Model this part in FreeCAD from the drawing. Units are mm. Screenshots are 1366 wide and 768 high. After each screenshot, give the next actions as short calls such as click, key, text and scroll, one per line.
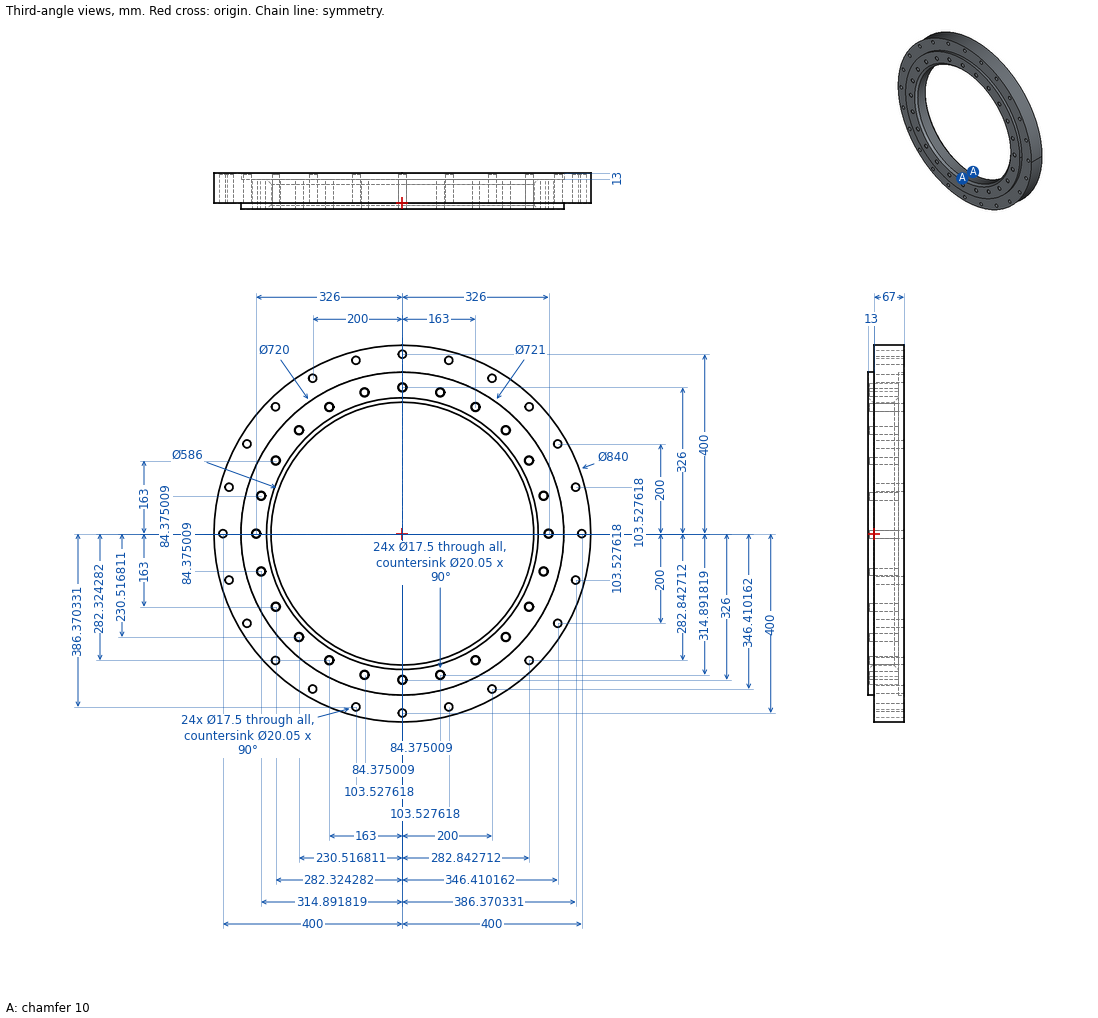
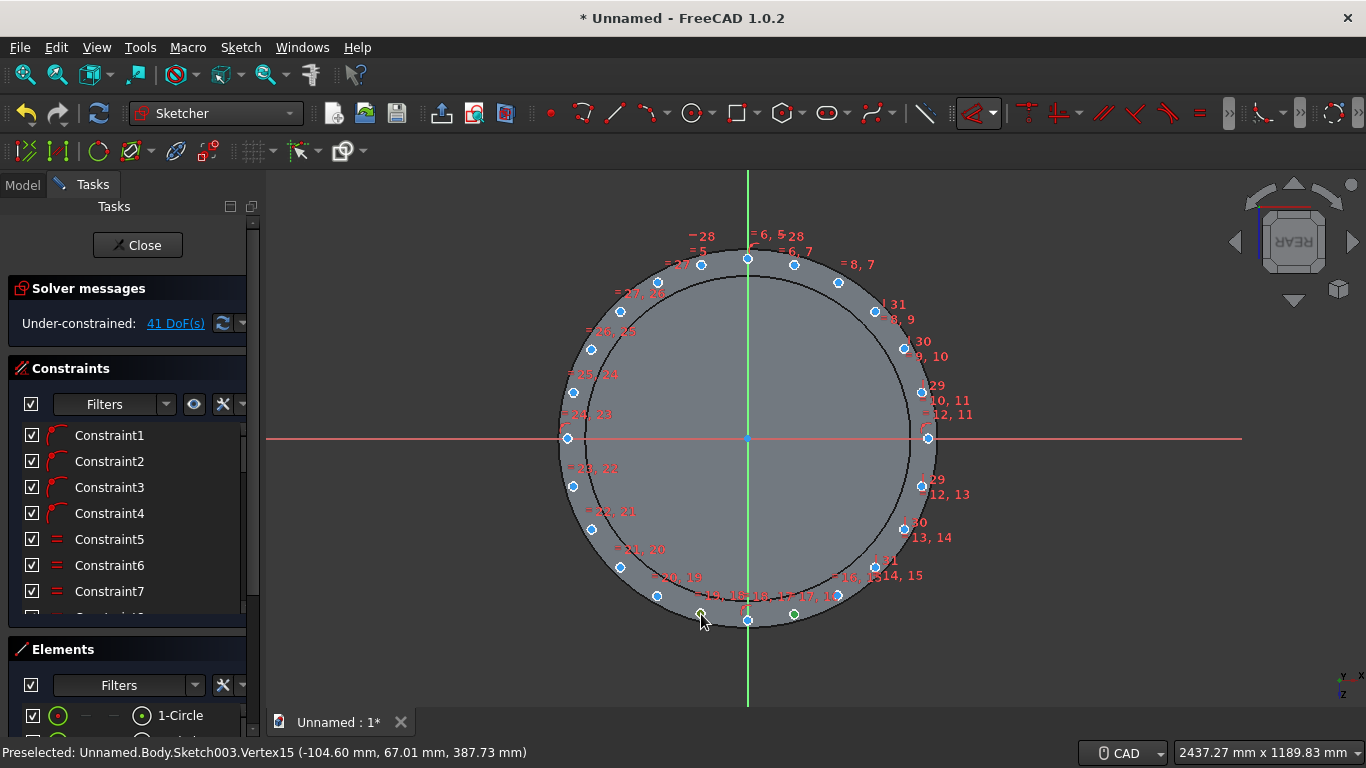
click(1082, 114)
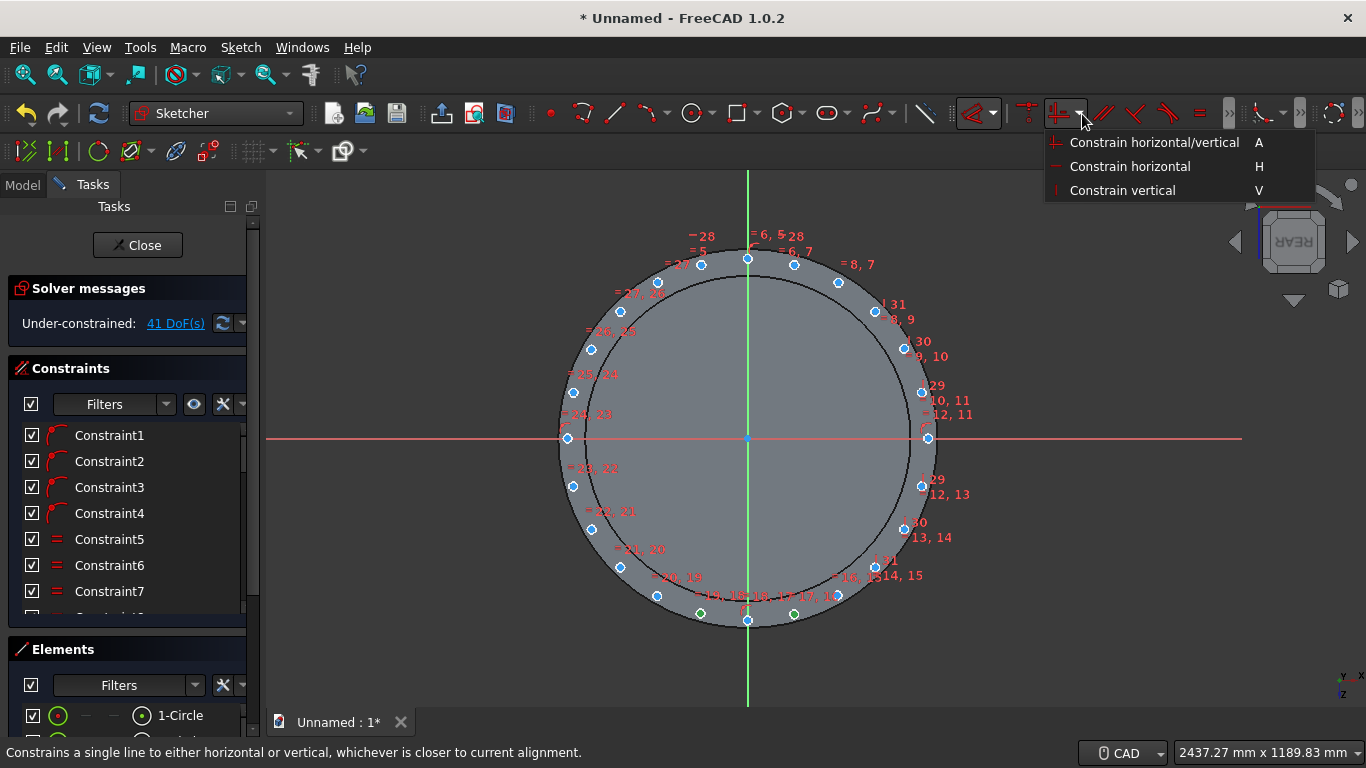
click(1180, 166)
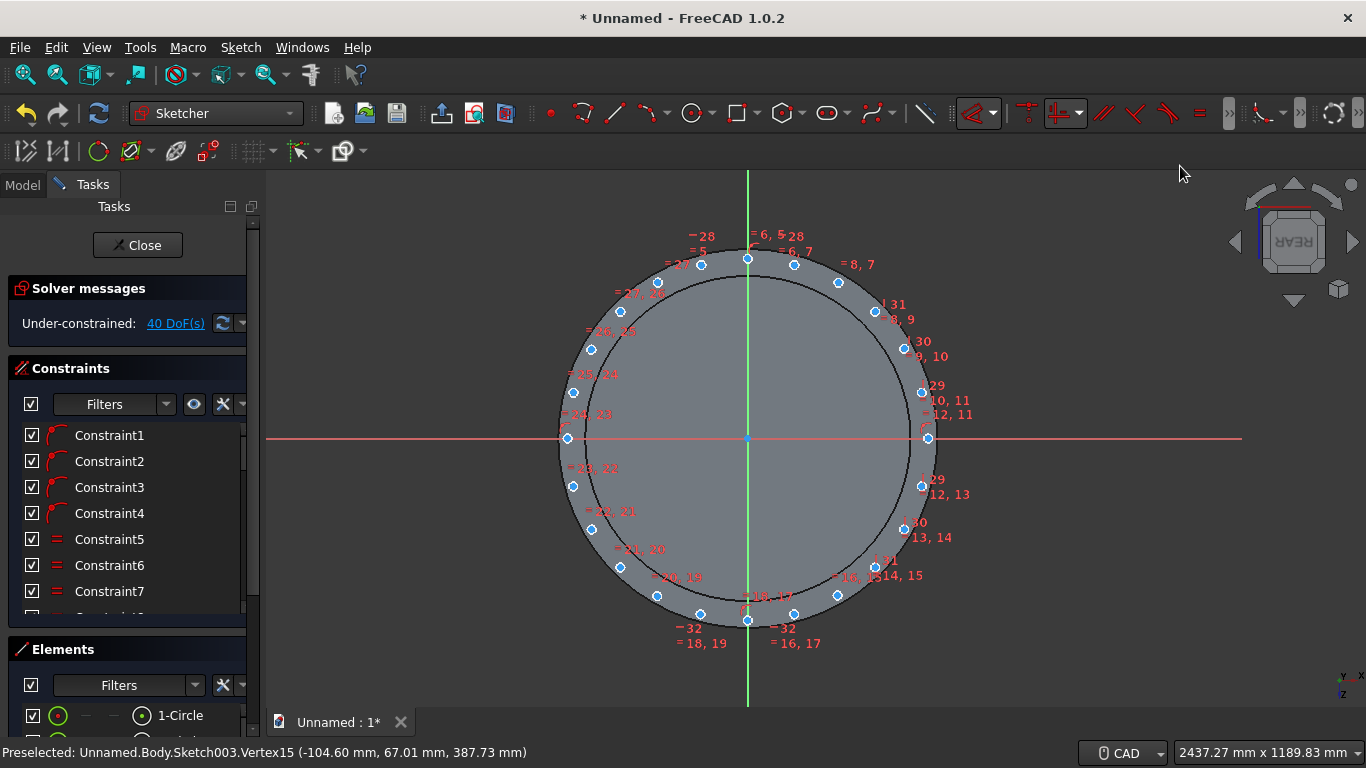
click(838, 596)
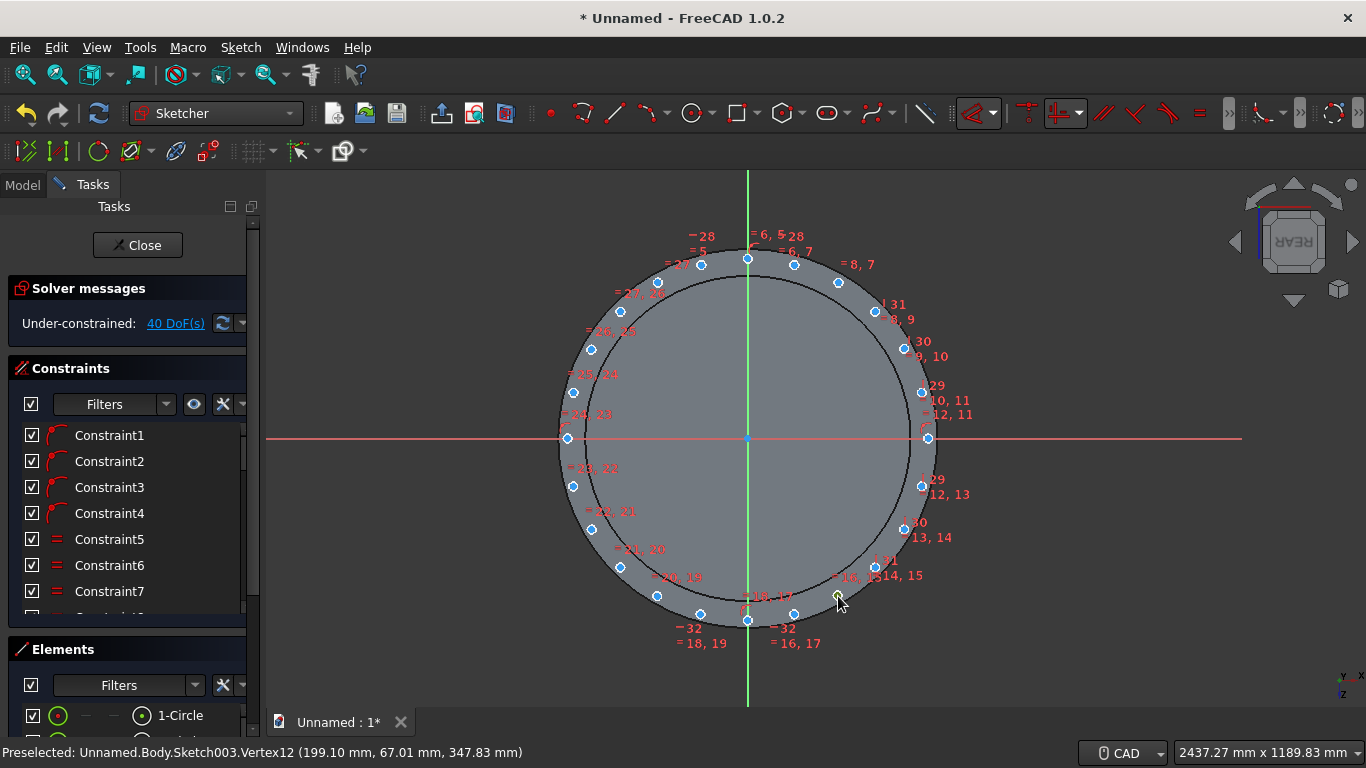
click(657, 596)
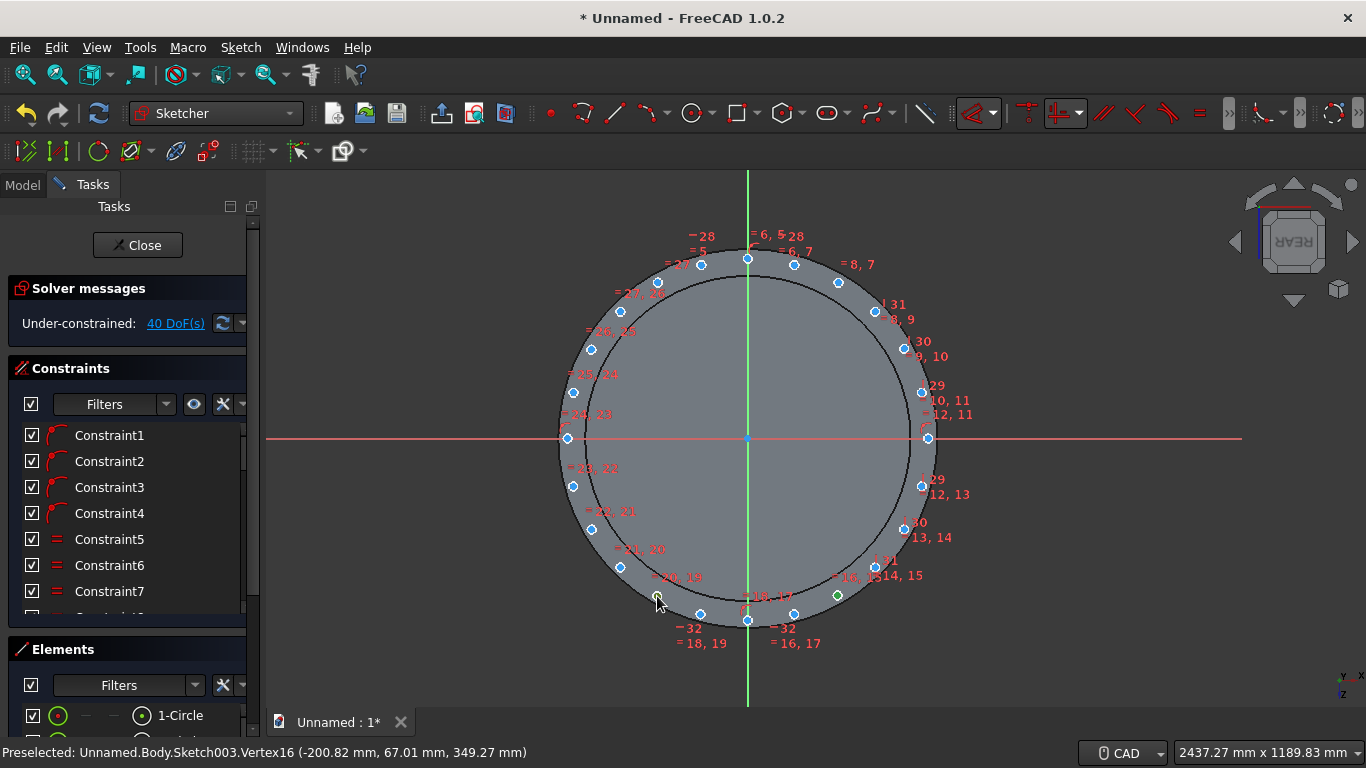
click(1082, 114)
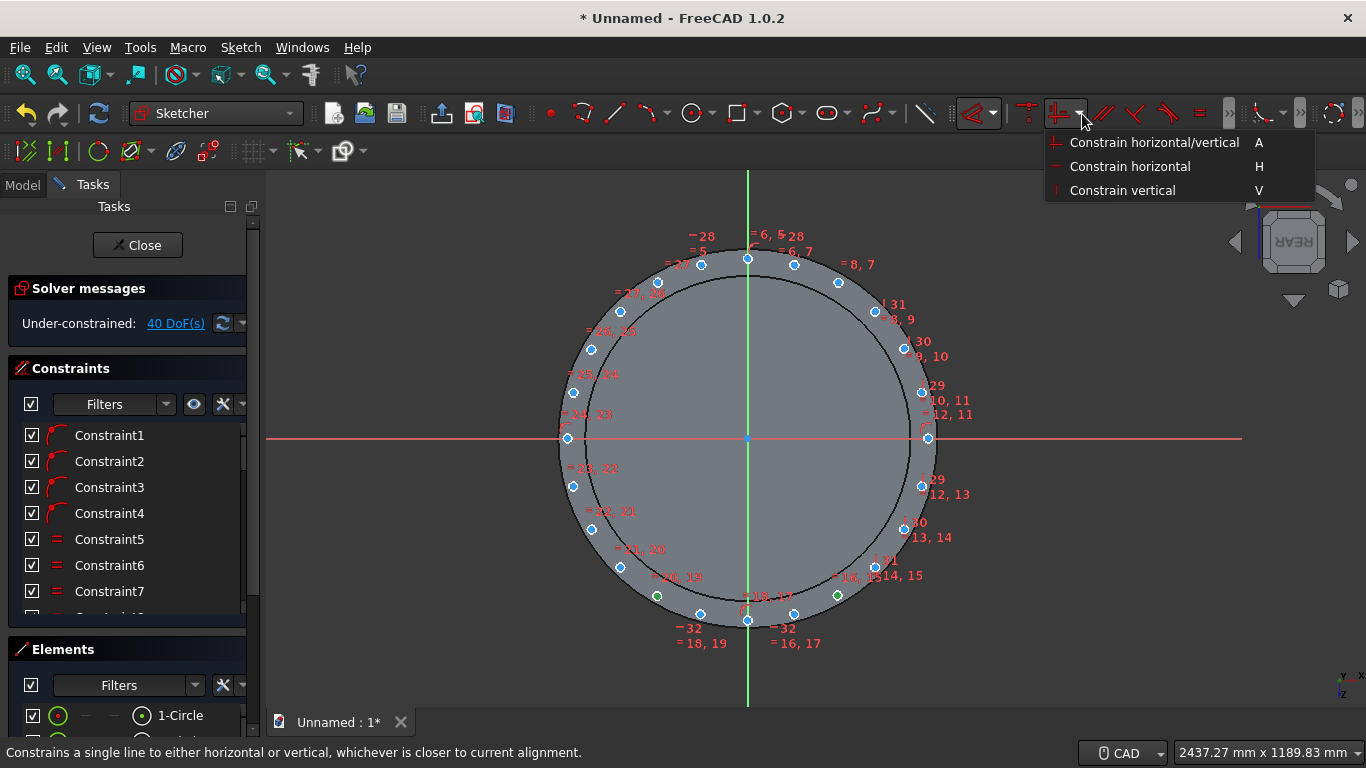
click(1180, 166)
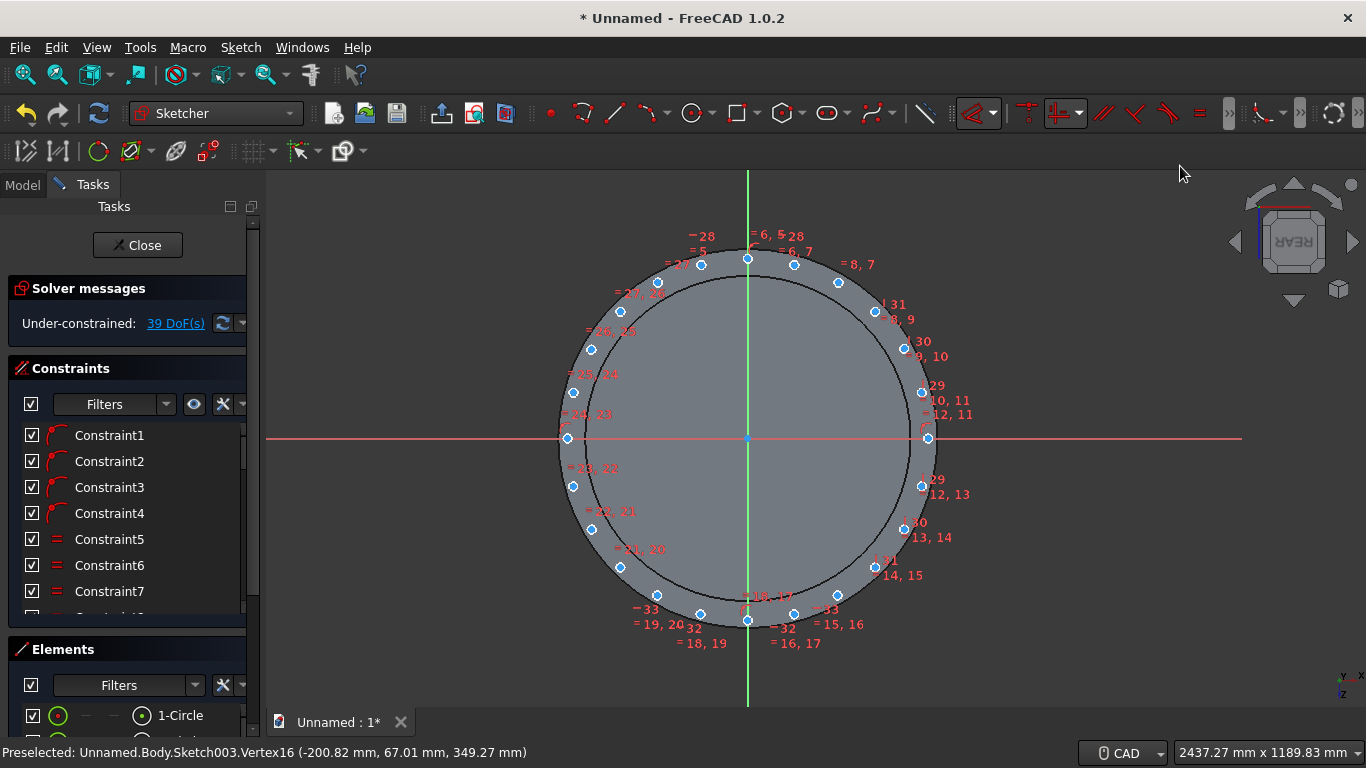
scroll(875, 568, up, 4)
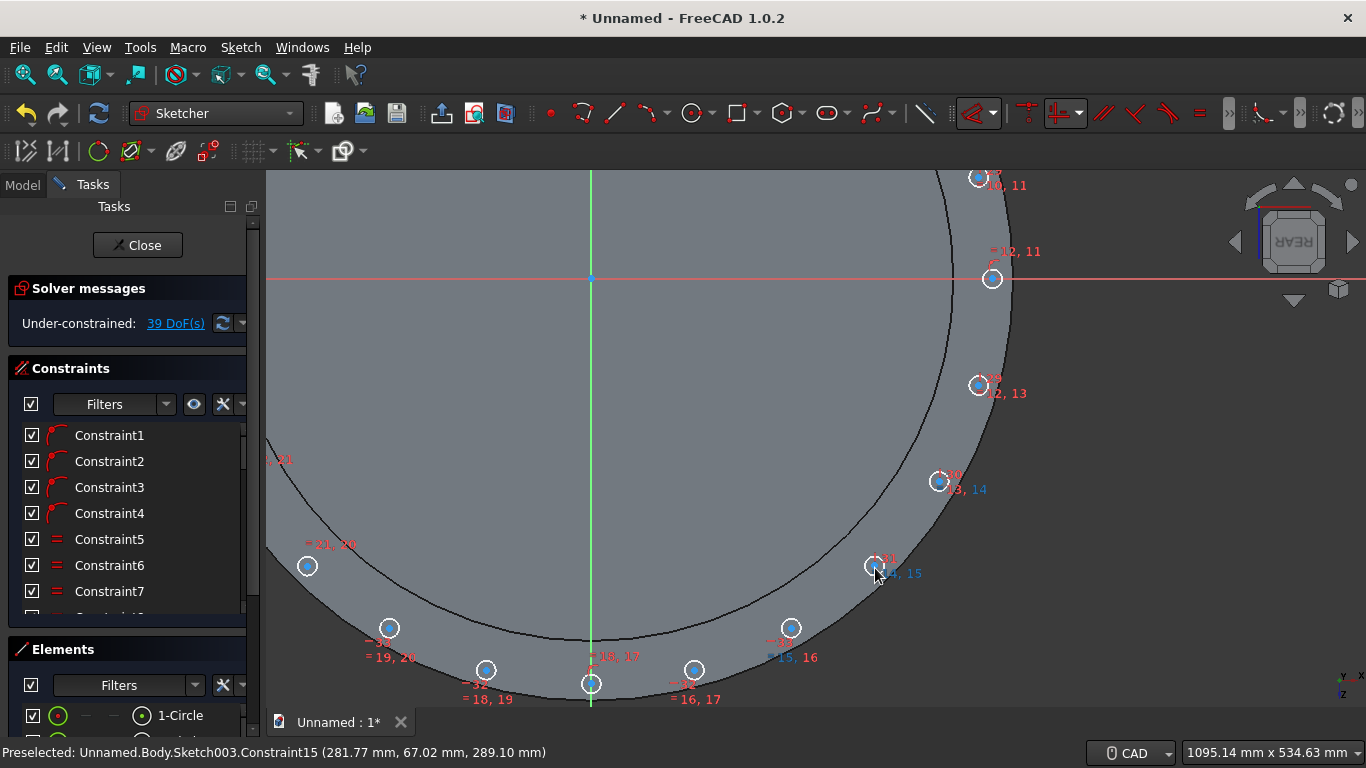
scroll(874, 566, up, 4)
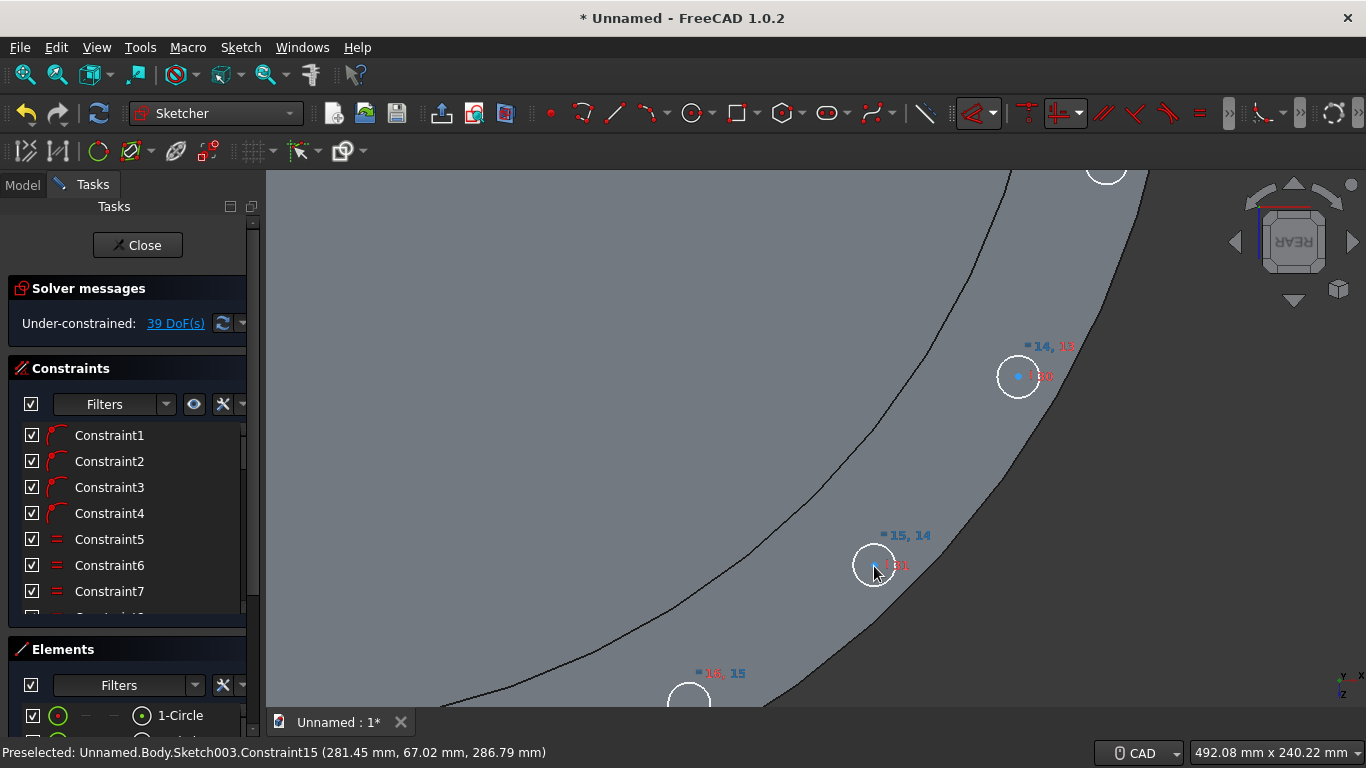
click(874, 565)